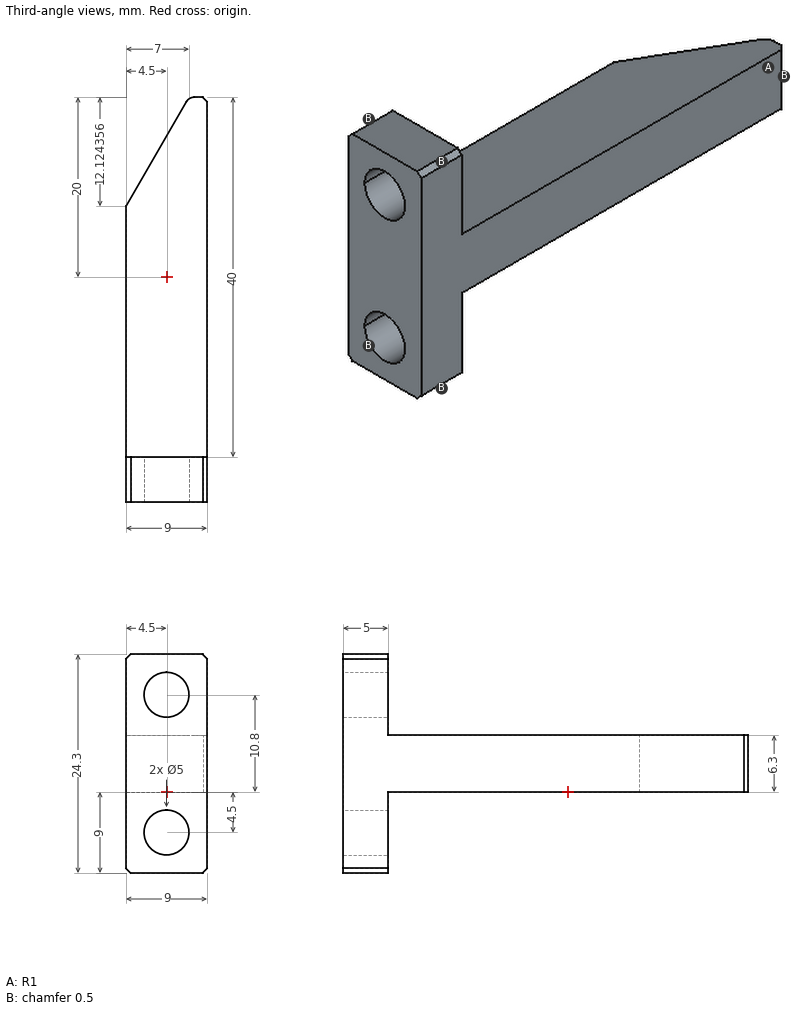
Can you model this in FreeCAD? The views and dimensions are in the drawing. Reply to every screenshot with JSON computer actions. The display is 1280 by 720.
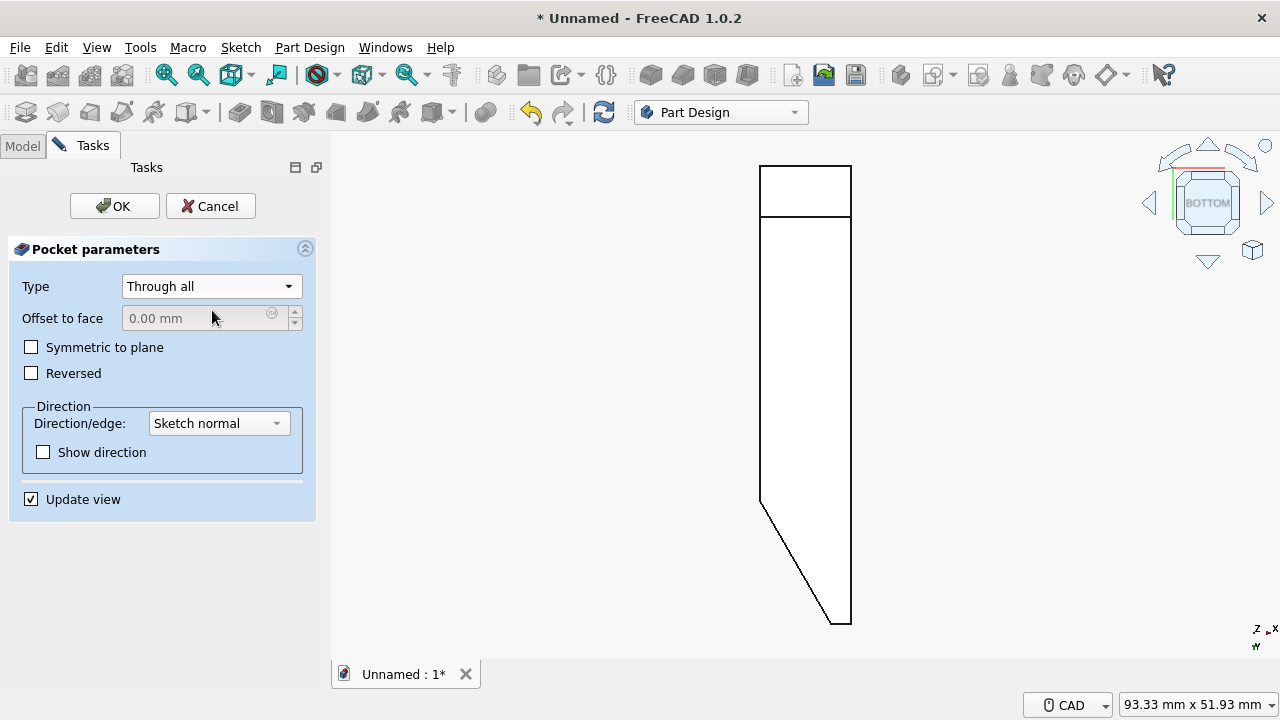
{"action": "left_click", "coordinate": [115, 206]}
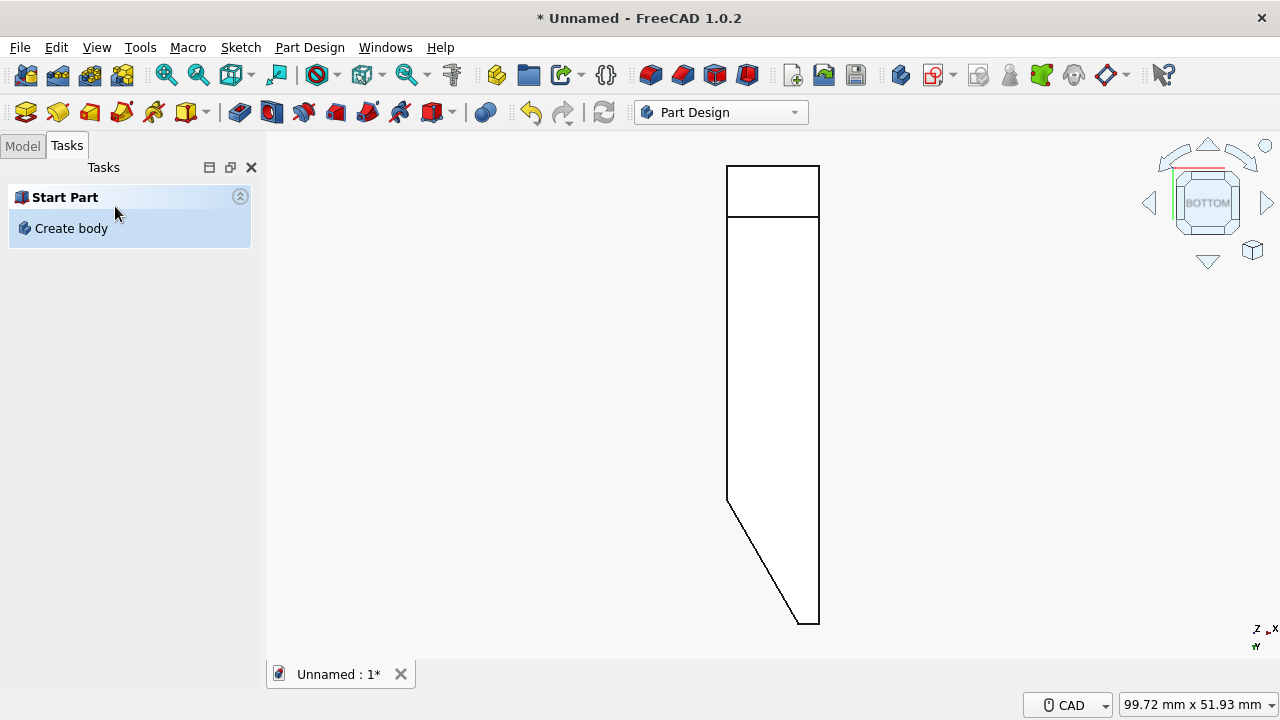
{"action": "key", "text": "4"}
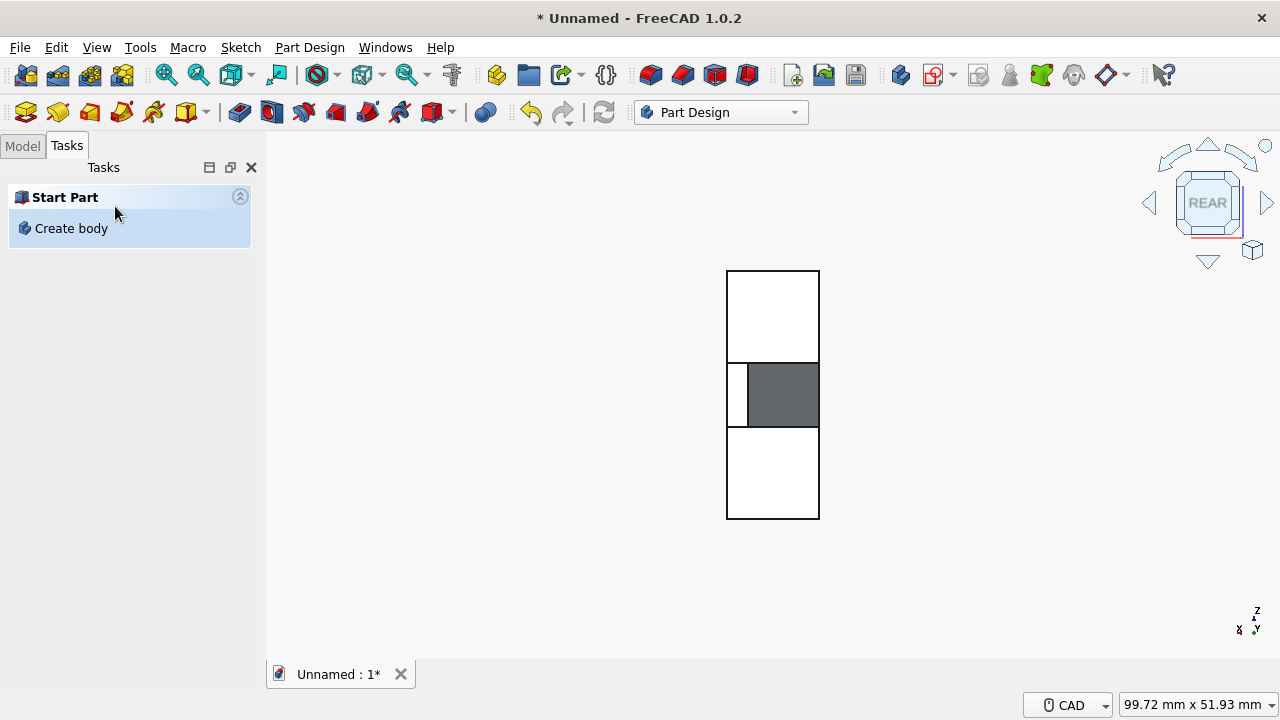
{"action": "left_click", "coordinate": [773, 316]}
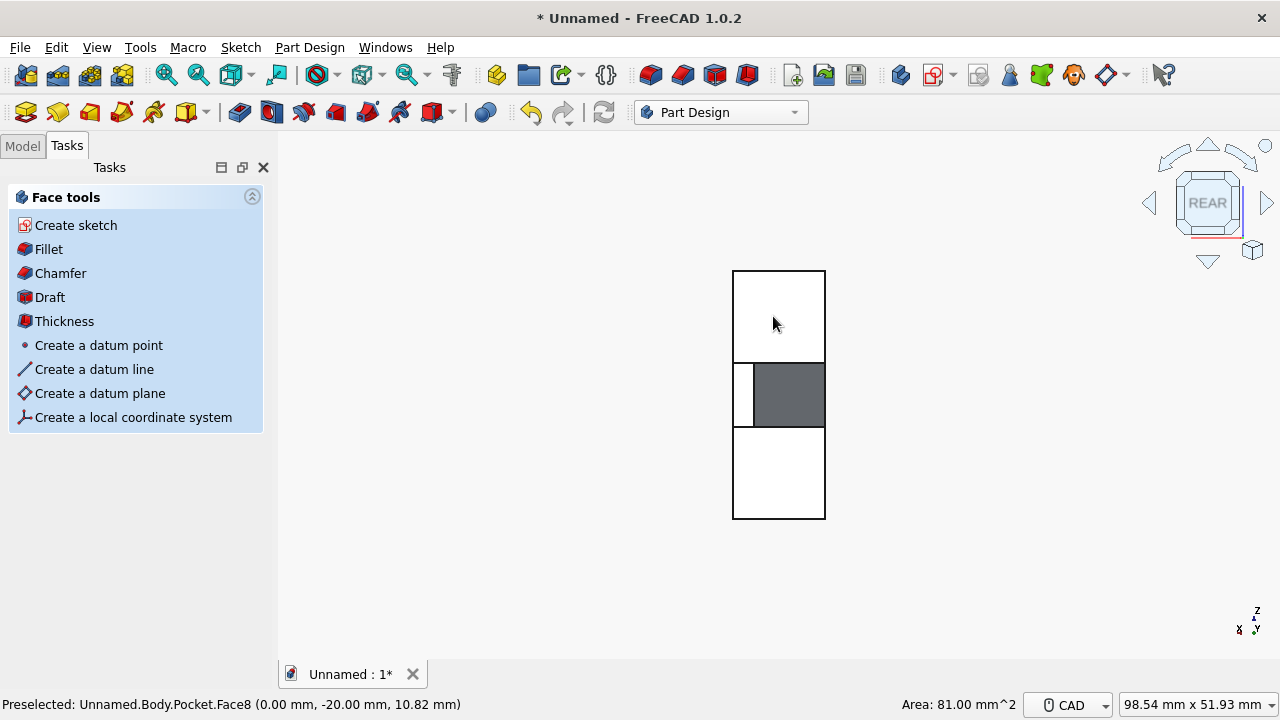
{"action": "left_click", "coordinate": [934, 76]}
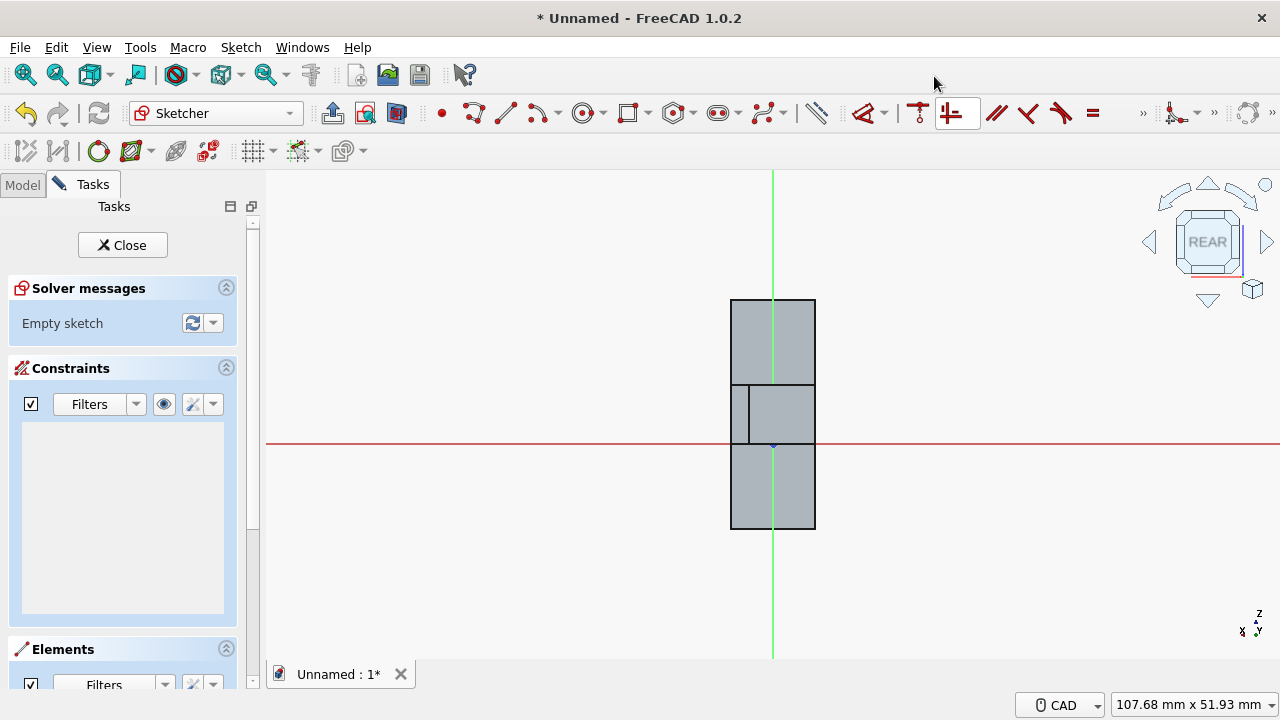
{"action": "key", "text": "q s"}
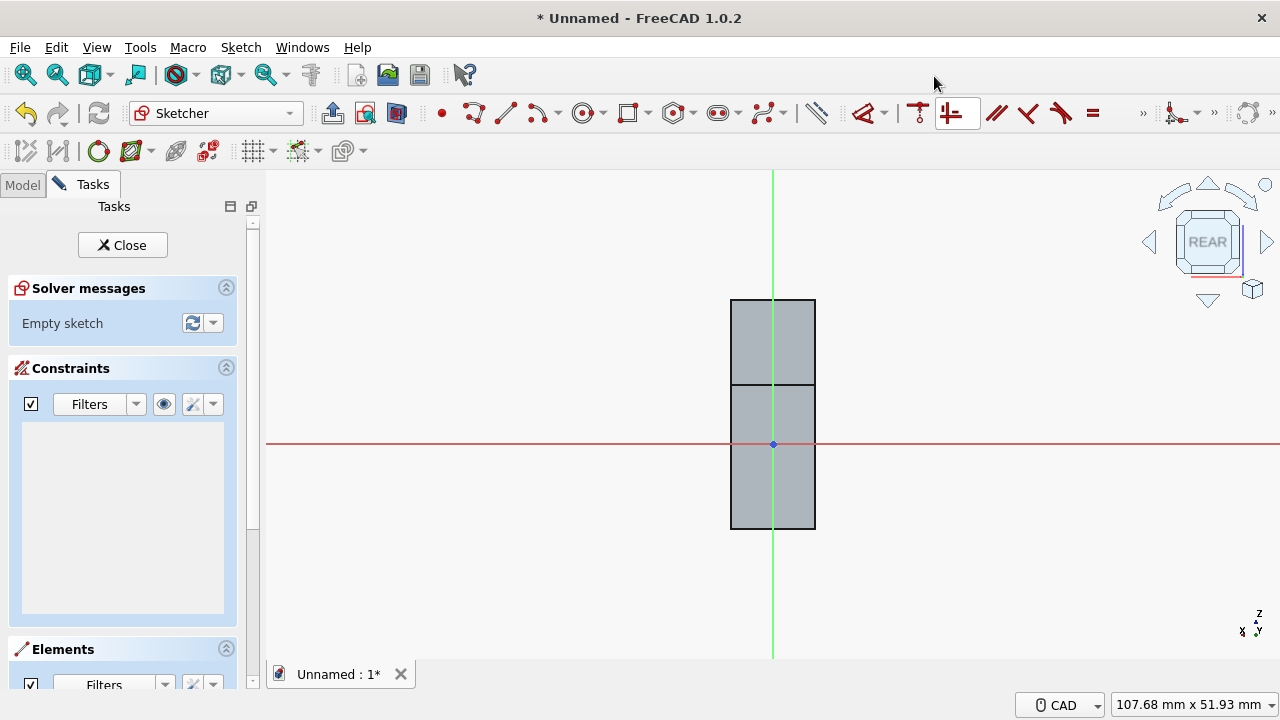
{"action": "scroll", "coordinate": [912, 414], "scroll_direction": "up", "scroll_amount": 2}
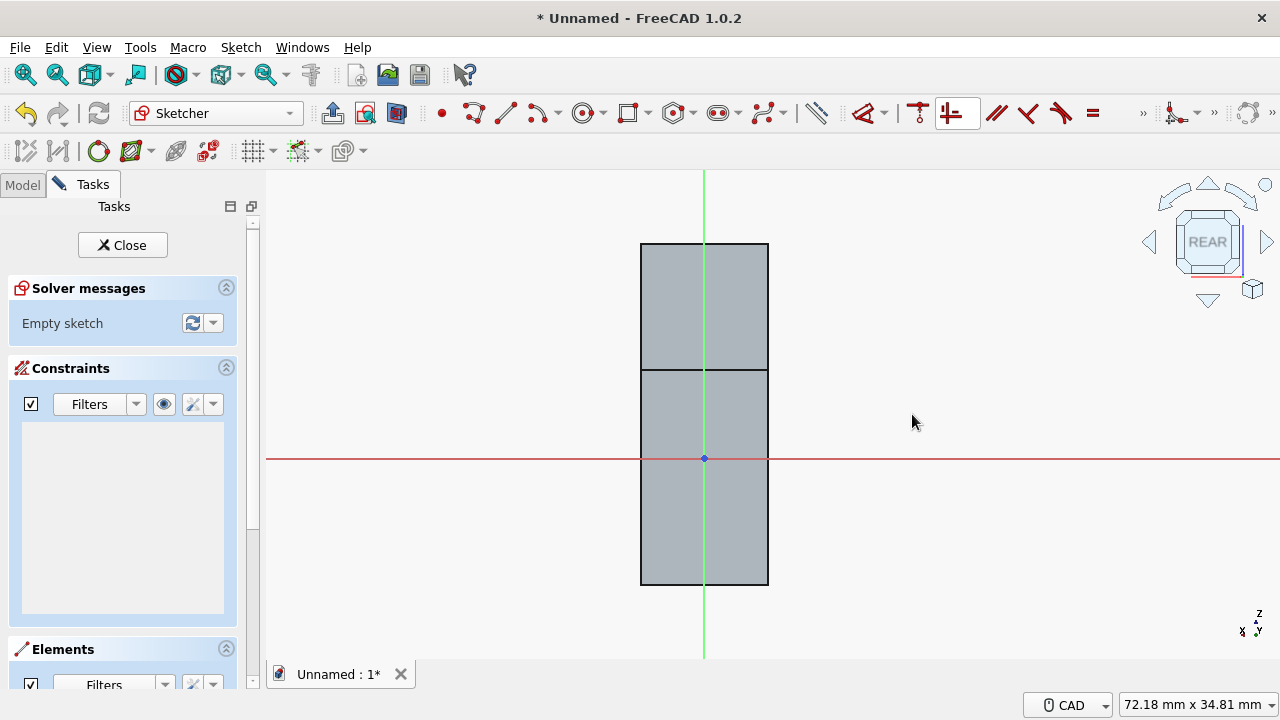
{"action": "left_click", "coordinate": [584, 114]}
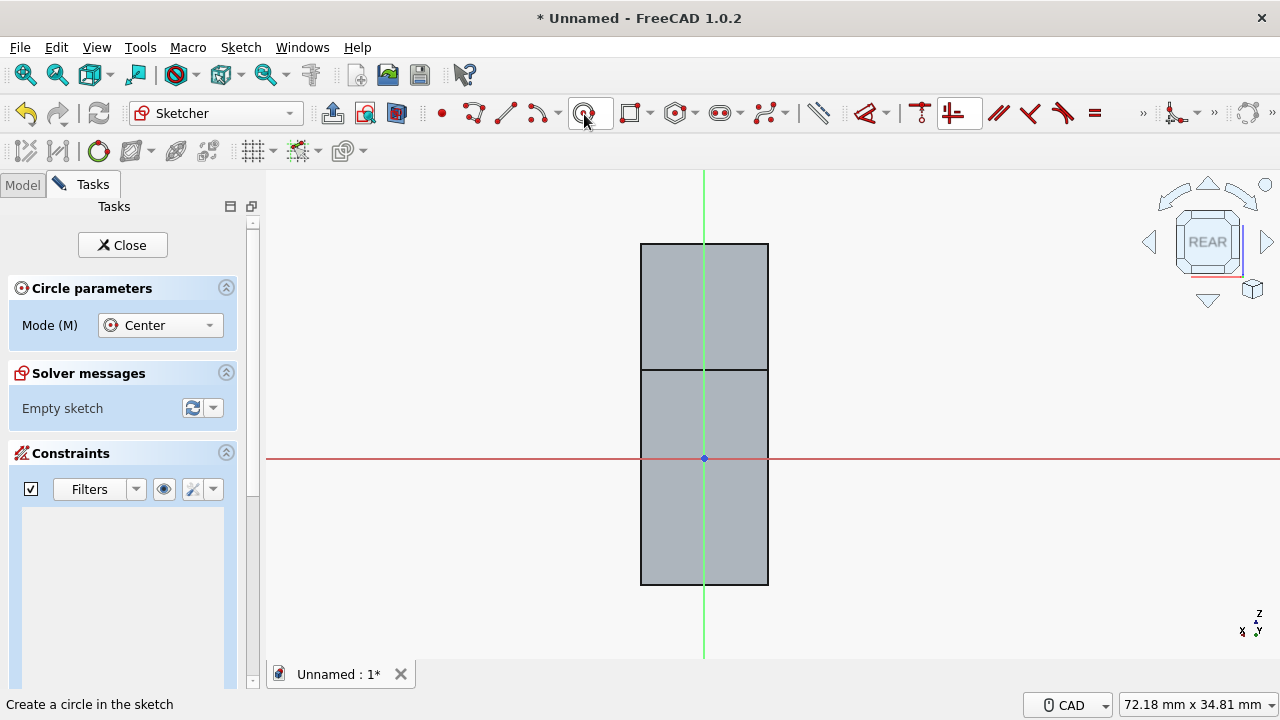
{"action": "left_click", "coordinate": [704, 522]}
{"action": "left_click", "coordinate": [729, 497]}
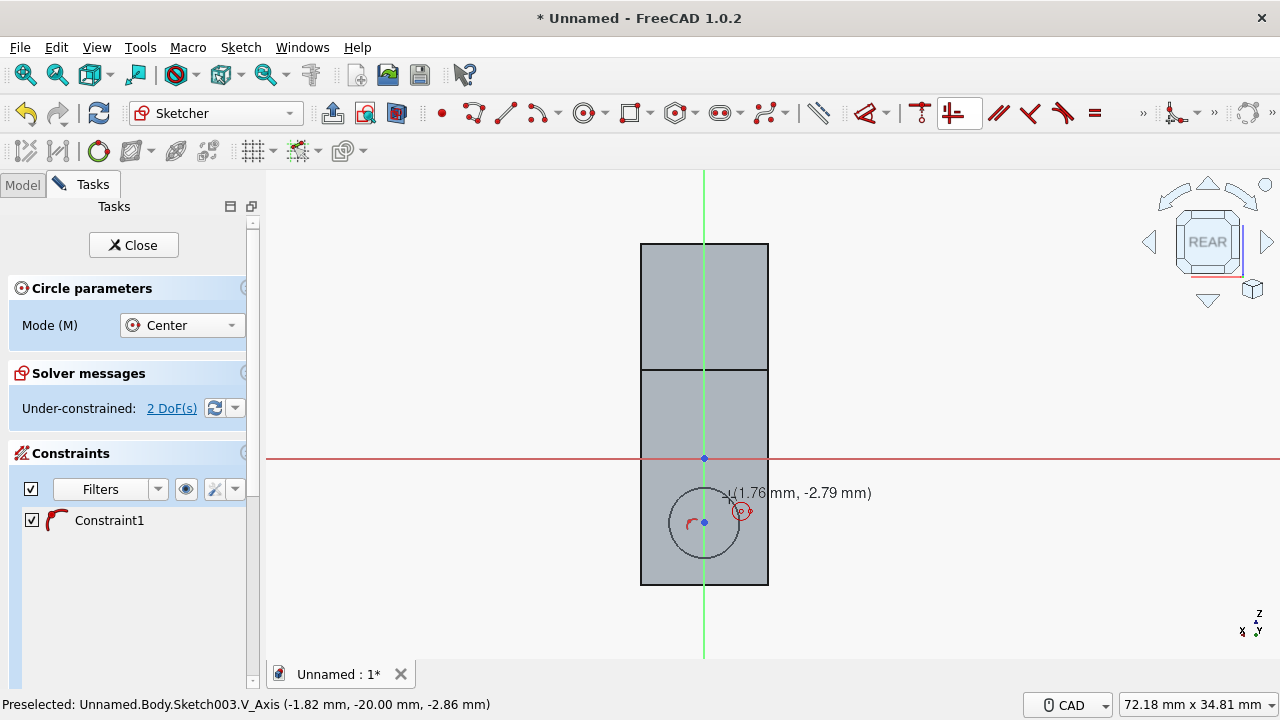
{"action": "left_click", "coordinate": [704, 307]}
{"action": "left_click", "coordinate": [729, 282]}
{"action": "key", "text": "Escape"}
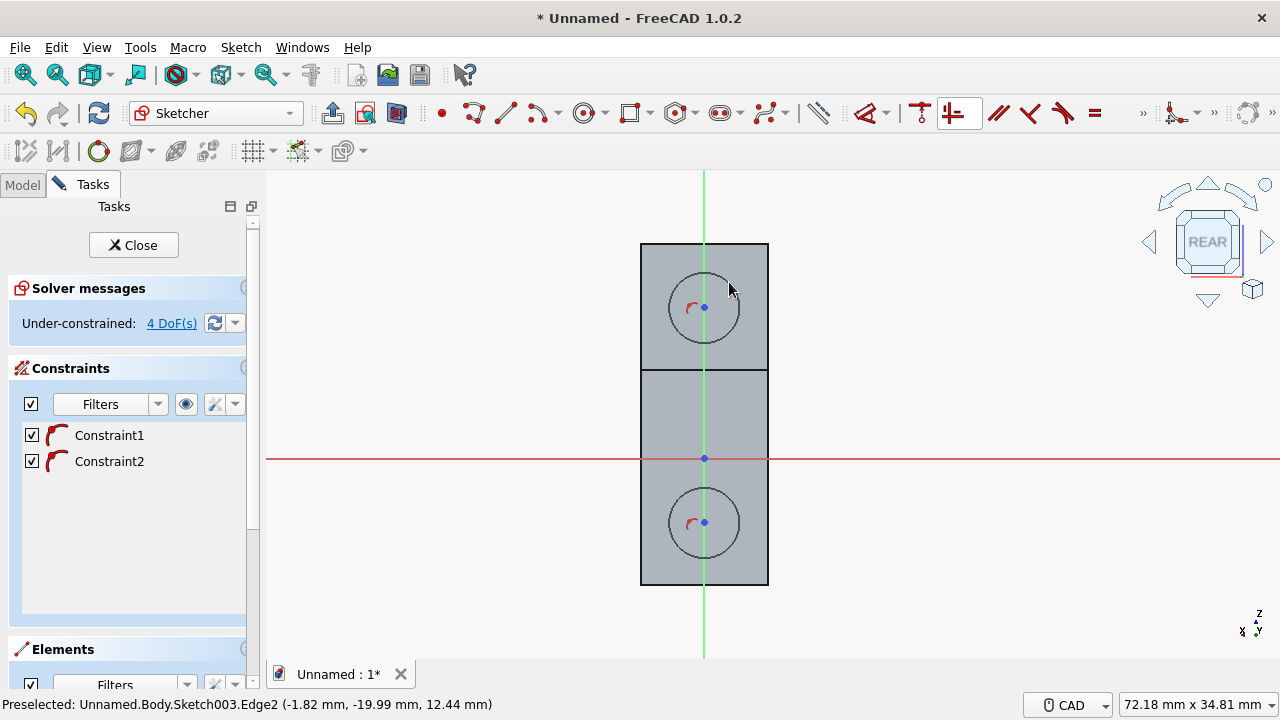
{"action": "left_click", "coordinate": [729, 498]}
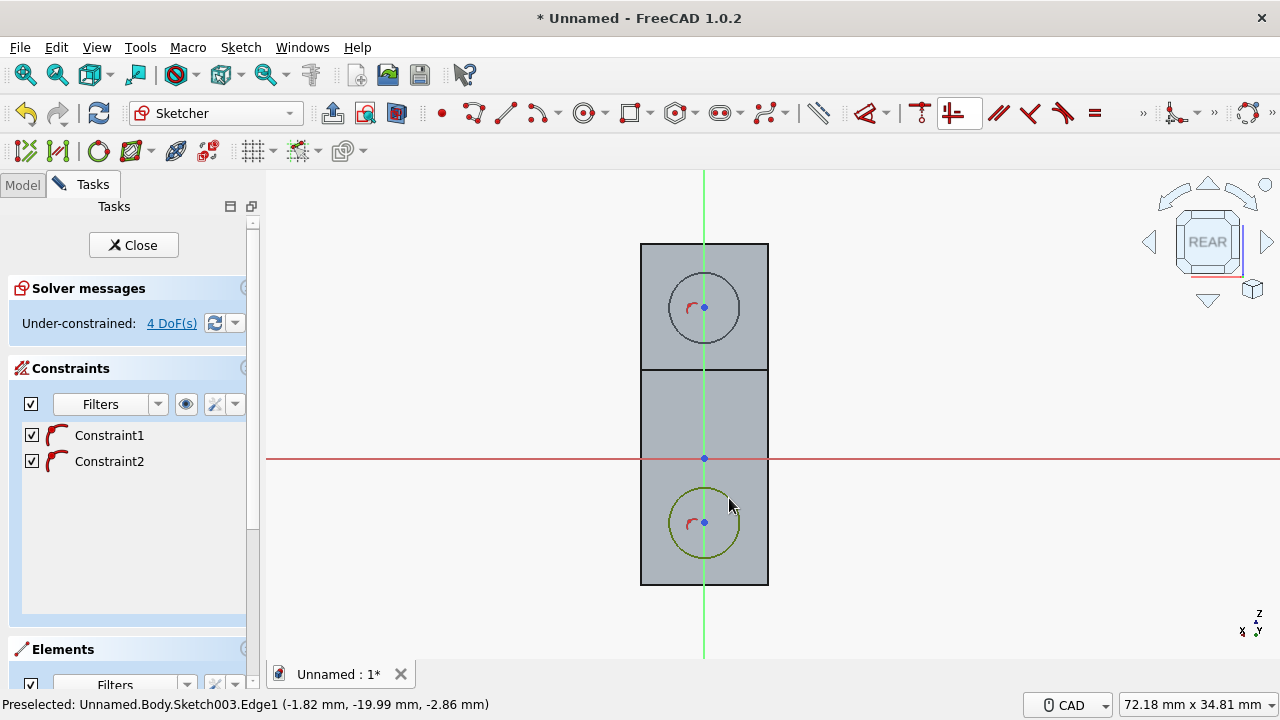
{"action": "left_click", "coordinate": [729, 283]}